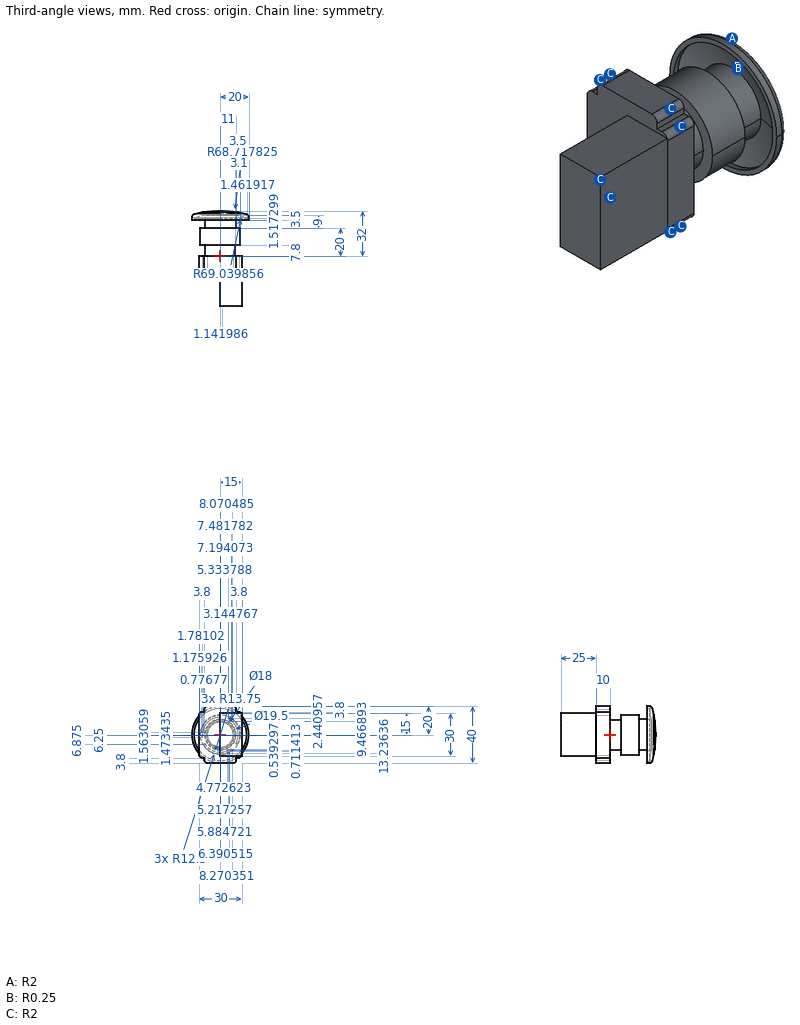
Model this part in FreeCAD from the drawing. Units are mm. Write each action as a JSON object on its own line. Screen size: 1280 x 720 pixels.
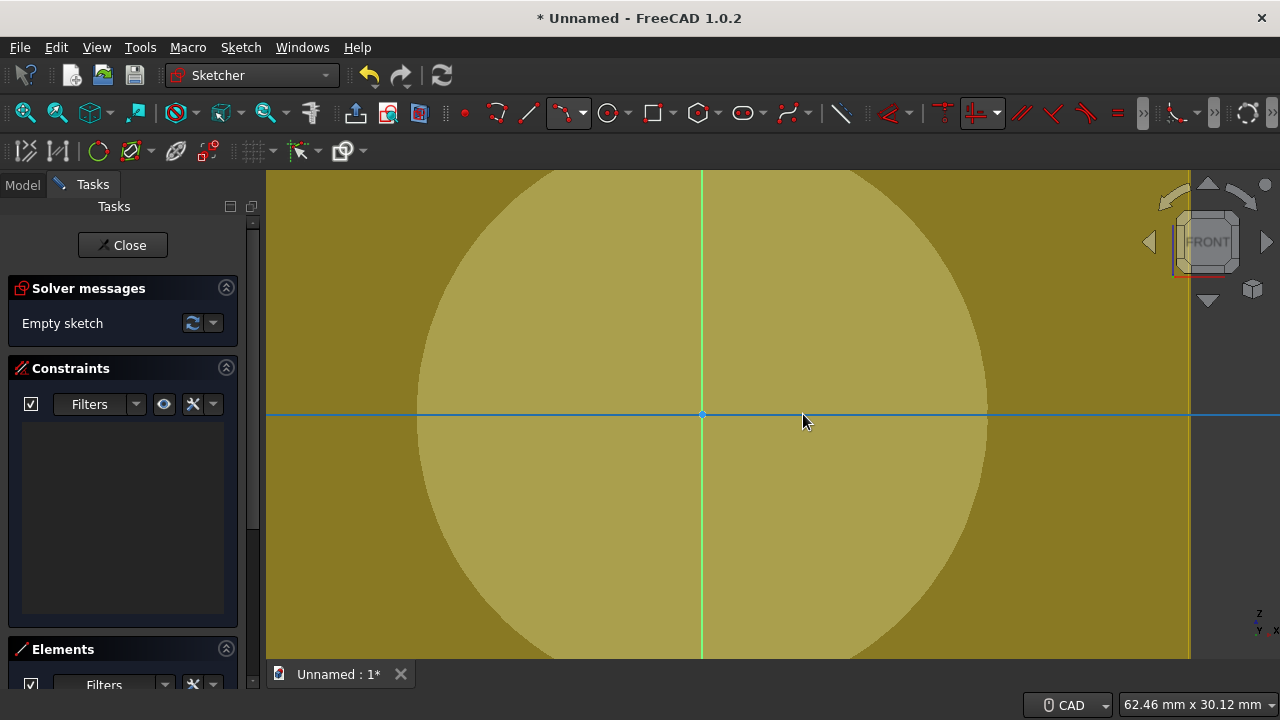
{"action": "left_click", "coordinate": [608, 114]}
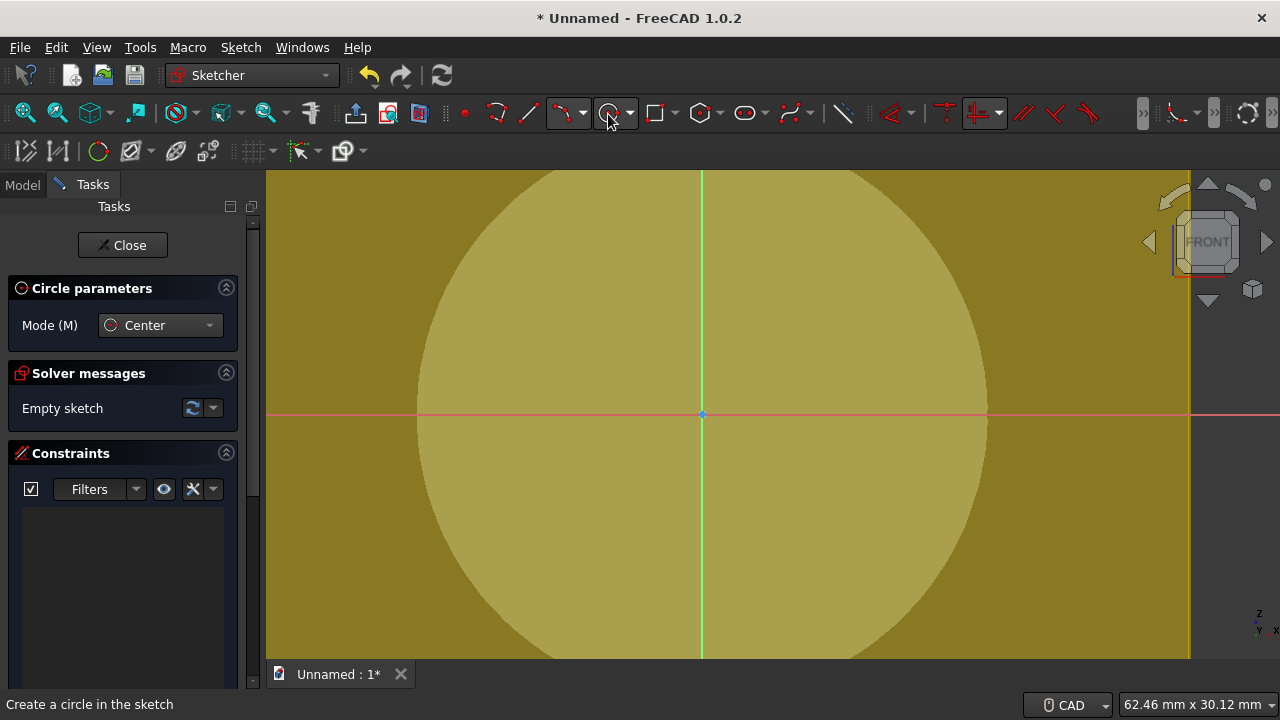
{"action": "left_click", "coordinate": [702, 414]}
{"action": "mouse_move", "coordinate": [814, 303]}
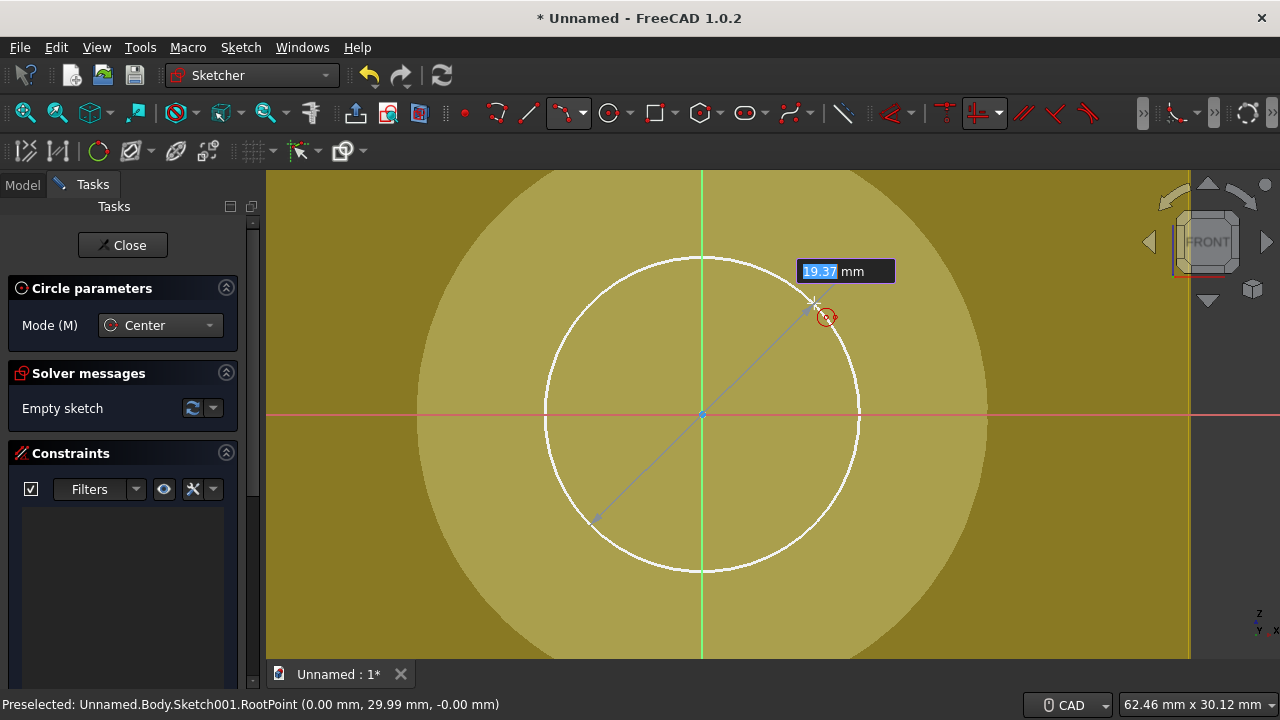
{"action": "type", "text": "19.5"}
{"action": "key", "text": "Return"}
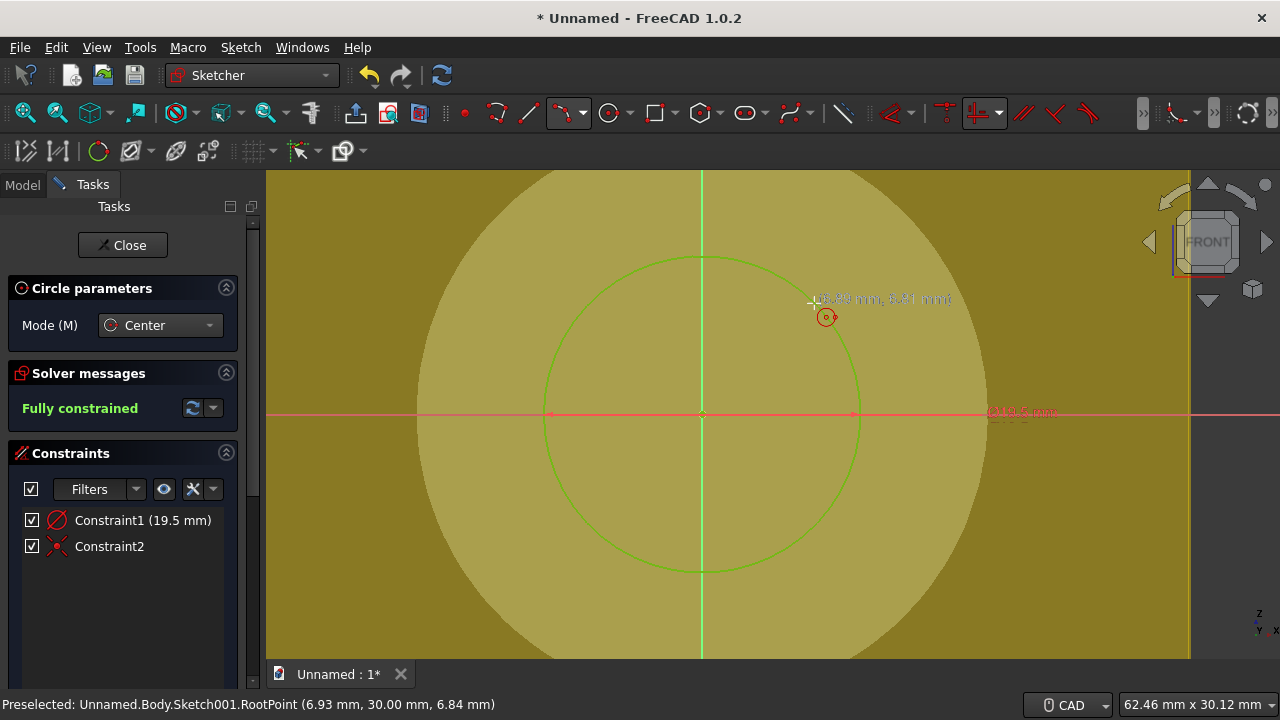
{"action": "left_click", "coordinate": [702, 414]}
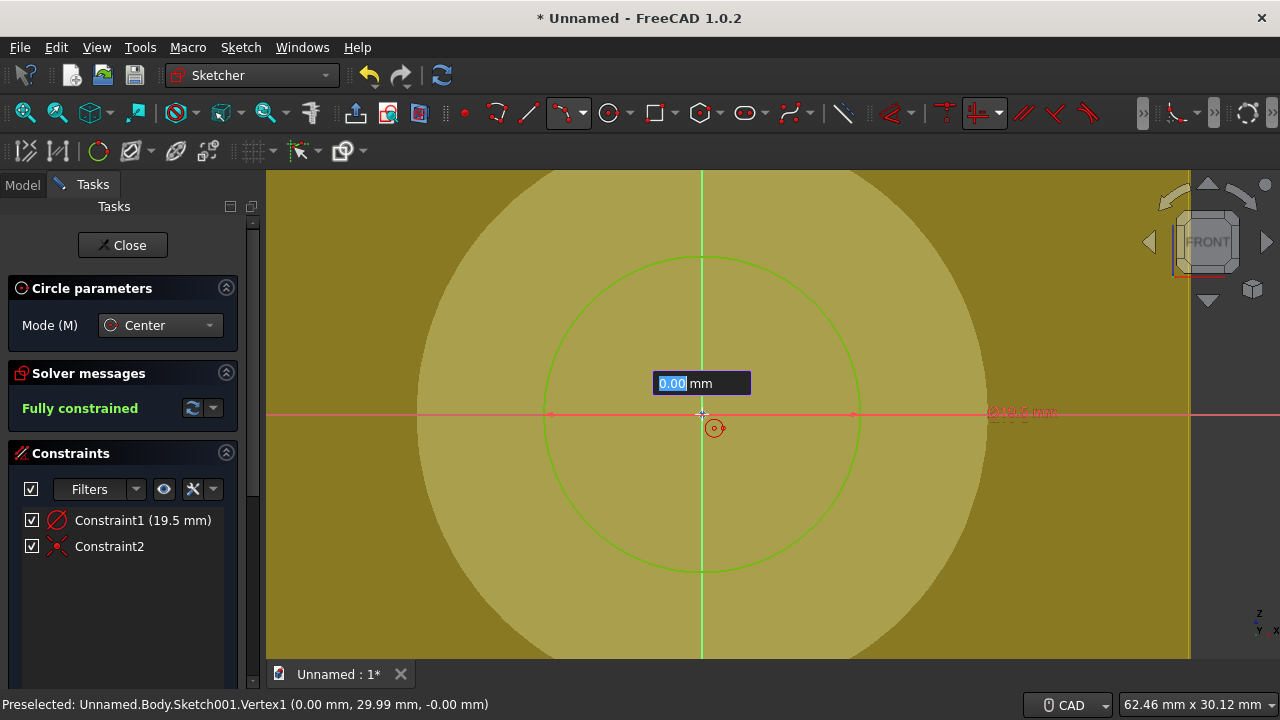
{"action": "scroll", "coordinate": [805, 311], "scroll_direction": "up", "scroll_amount": 2}
{"action": "mouse_move", "coordinate": [805, 311]}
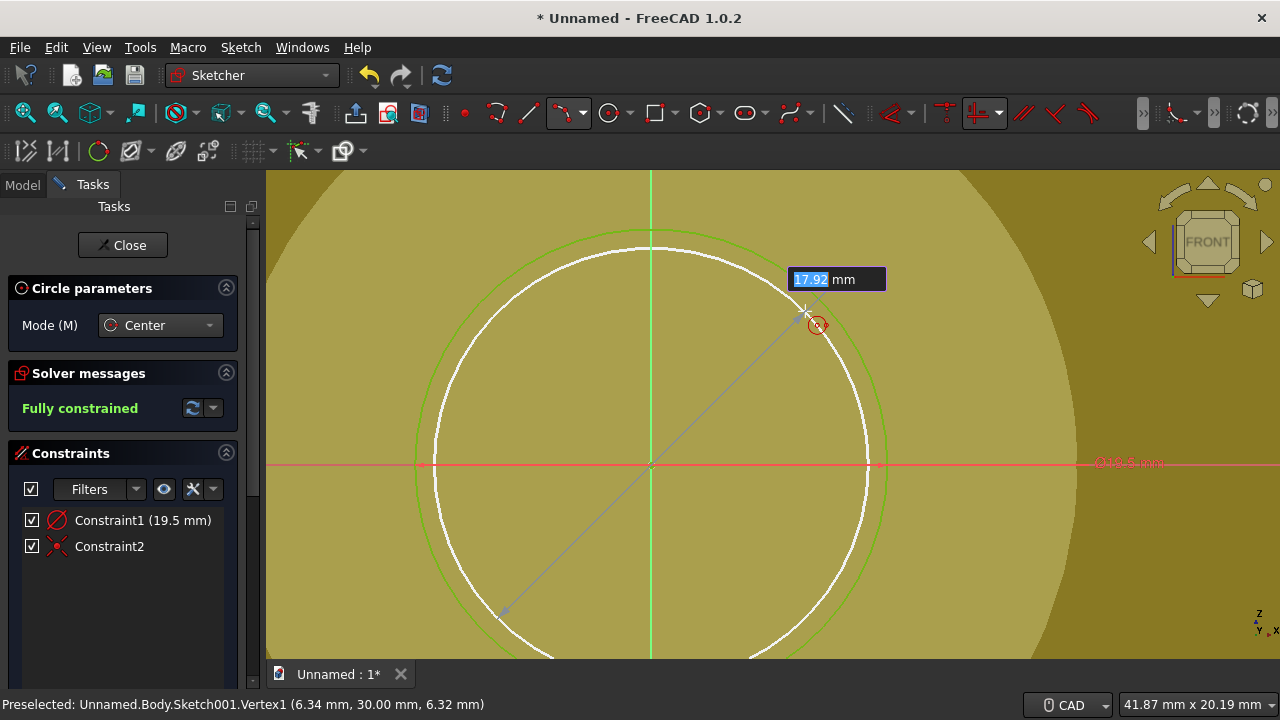
{"action": "type", "text": "18"}
{"action": "key", "text": "Return"}
{"action": "key", "text": "Escape"}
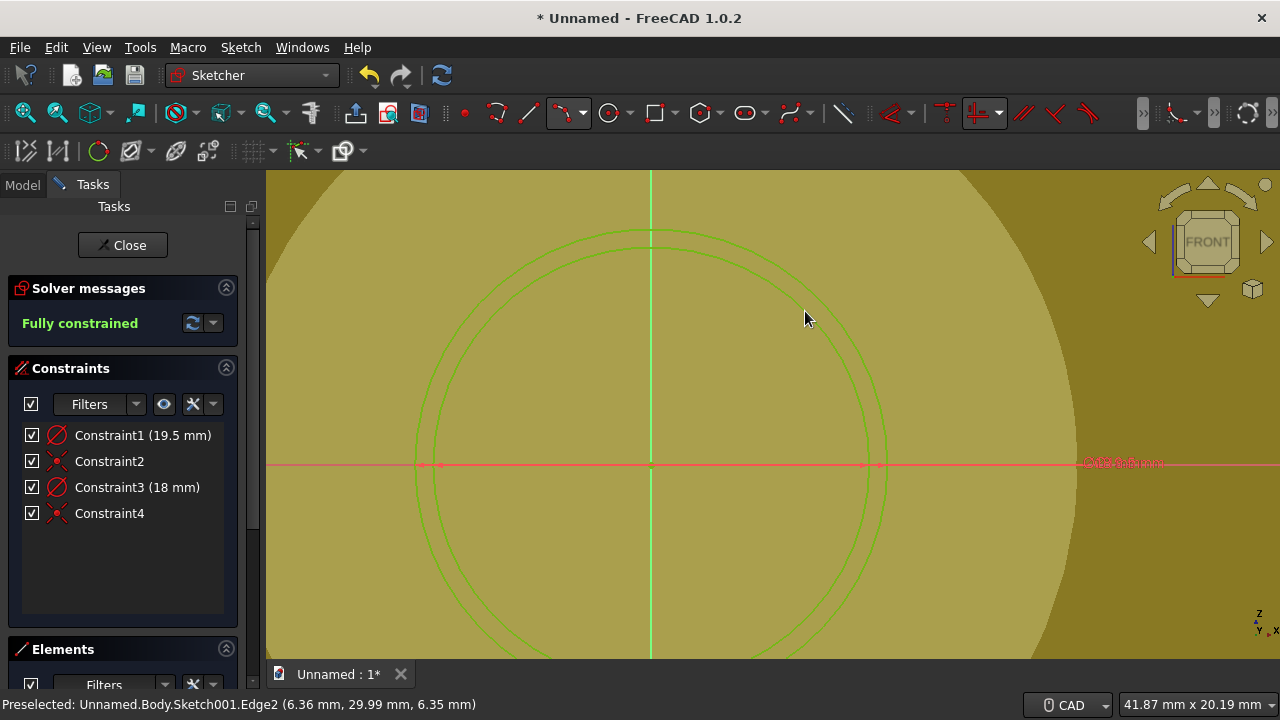
{"action": "left_click", "coordinate": [123, 245]}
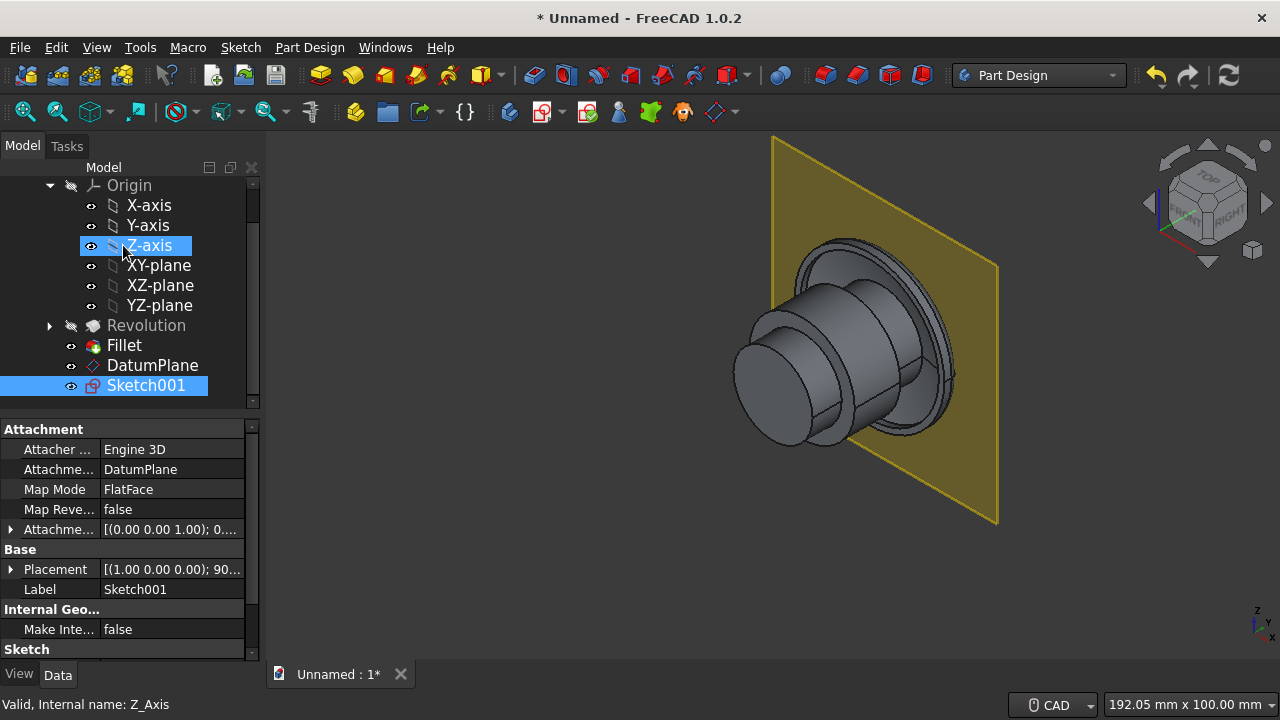
{"action": "left_click", "coordinate": [536, 76]}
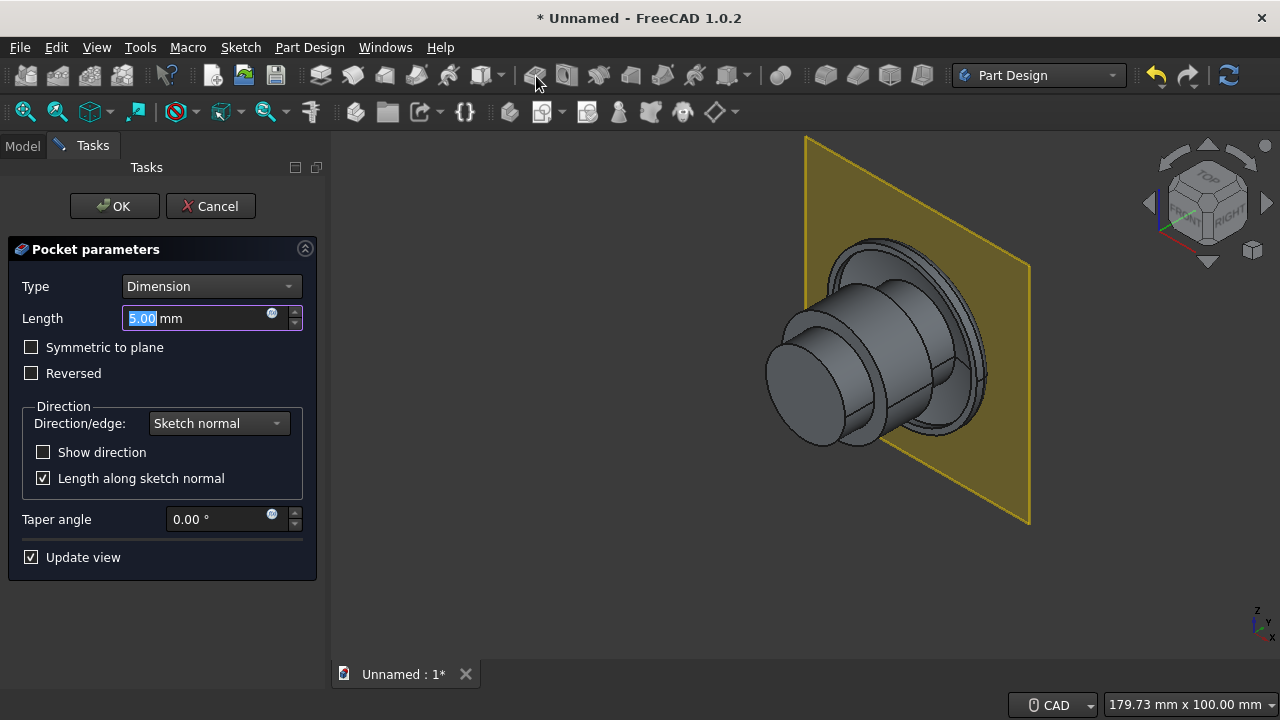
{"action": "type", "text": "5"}
{"action": "key", "text": "Tab"}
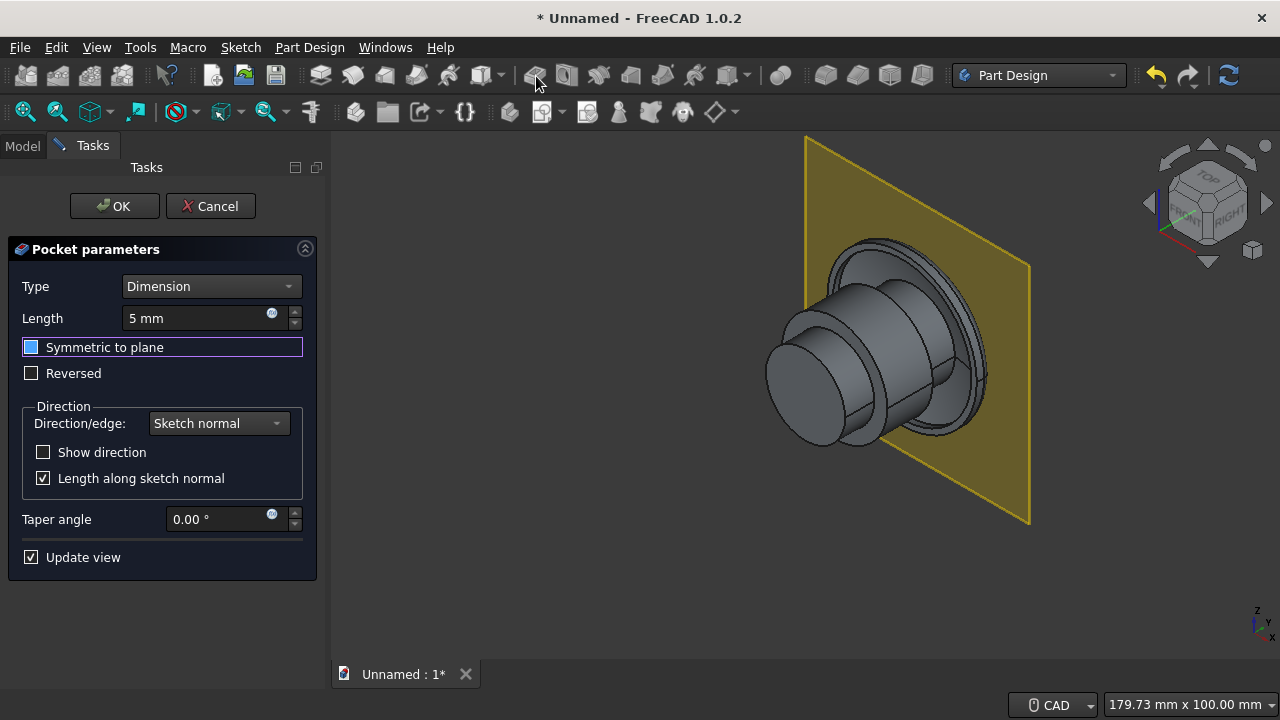
{"action": "left_click", "coordinate": [115, 206]}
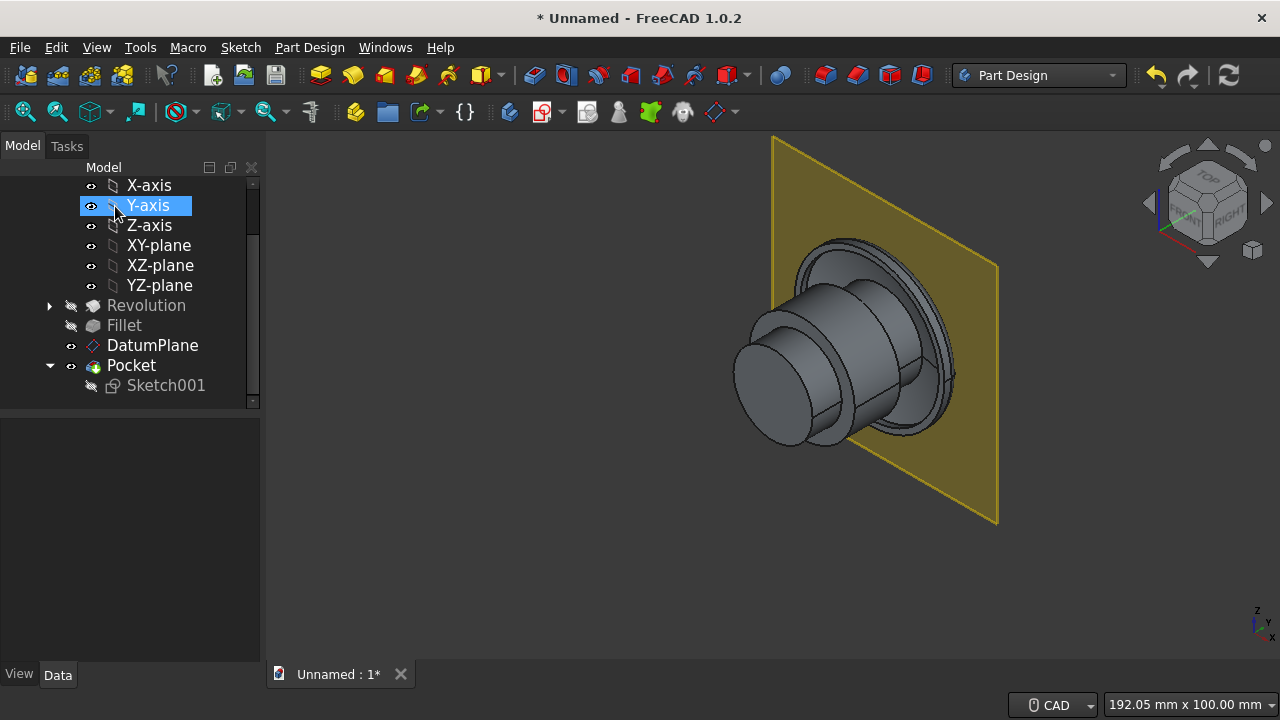
{"action": "left_click", "coordinate": [116, 346]}
{"action": "key", "text": "space"}